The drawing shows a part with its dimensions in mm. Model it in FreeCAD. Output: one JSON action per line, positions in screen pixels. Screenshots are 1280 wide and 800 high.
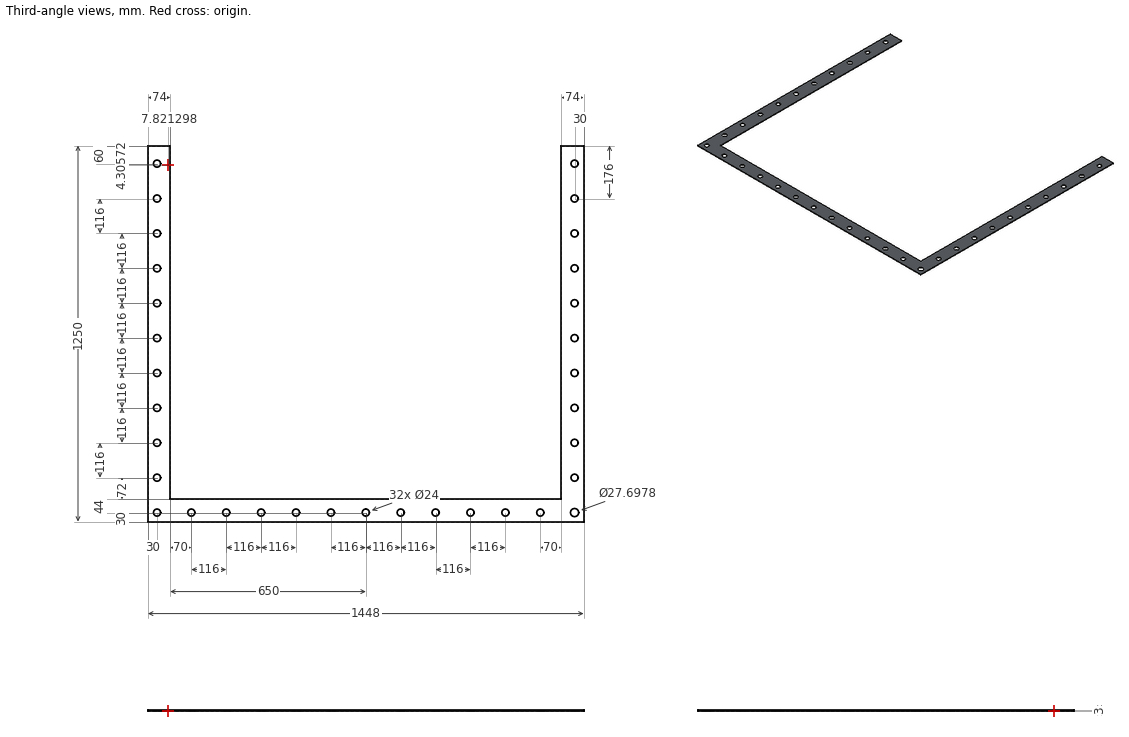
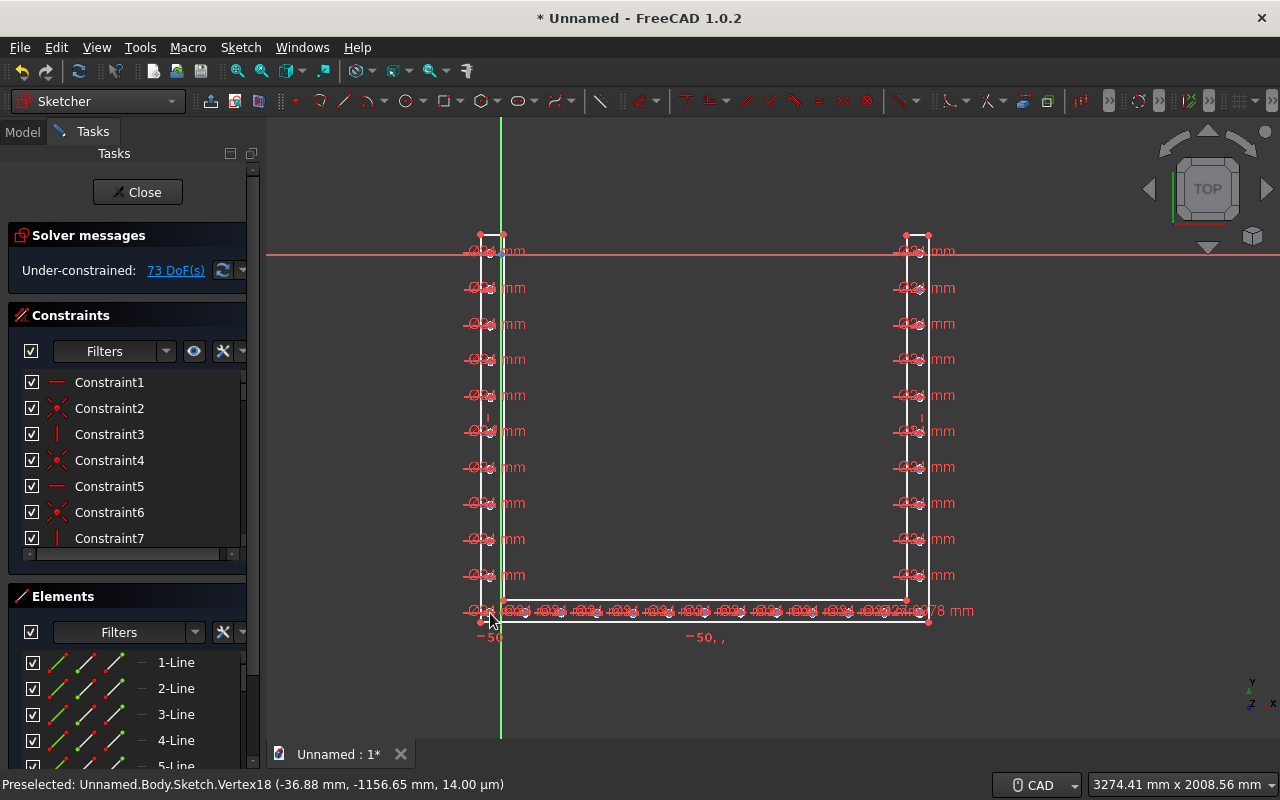
{"action": "left_click", "coordinate": [490, 577]}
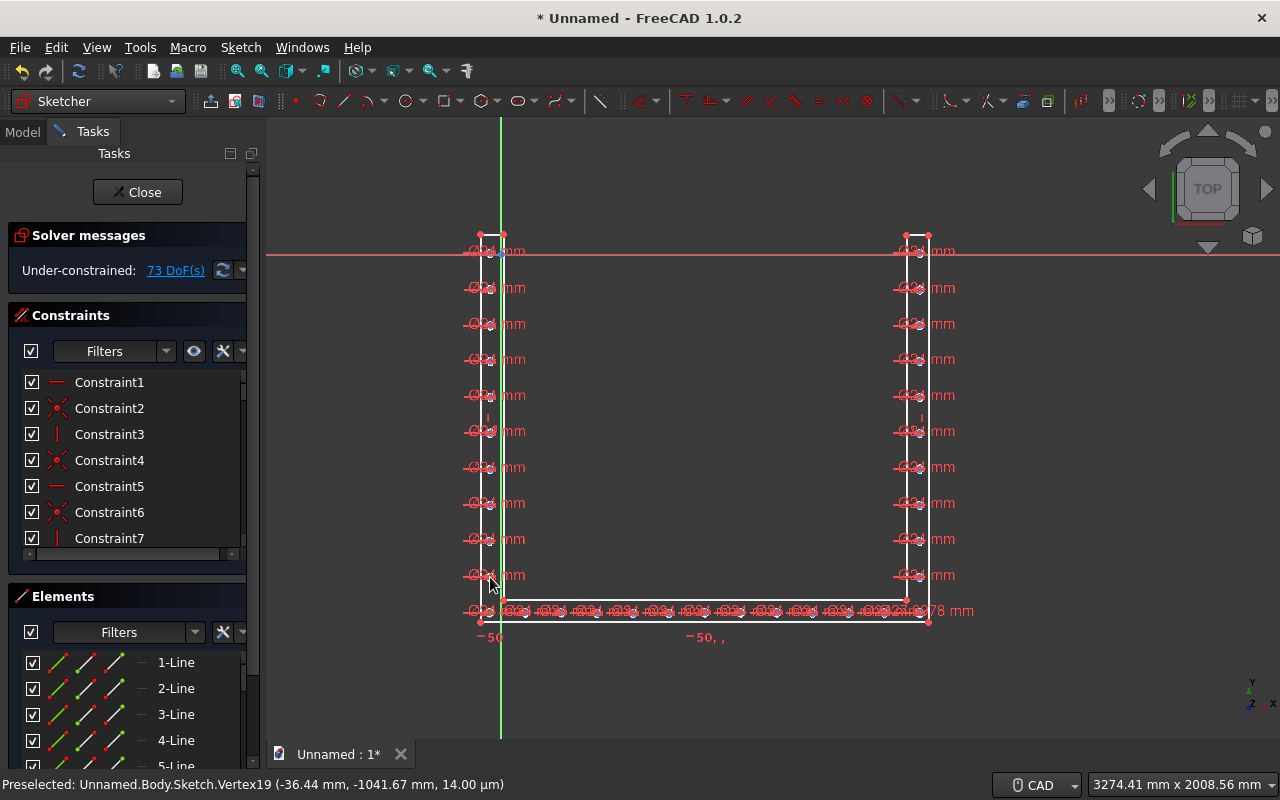
{"action": "left_click", "coordinate": [728, 102]}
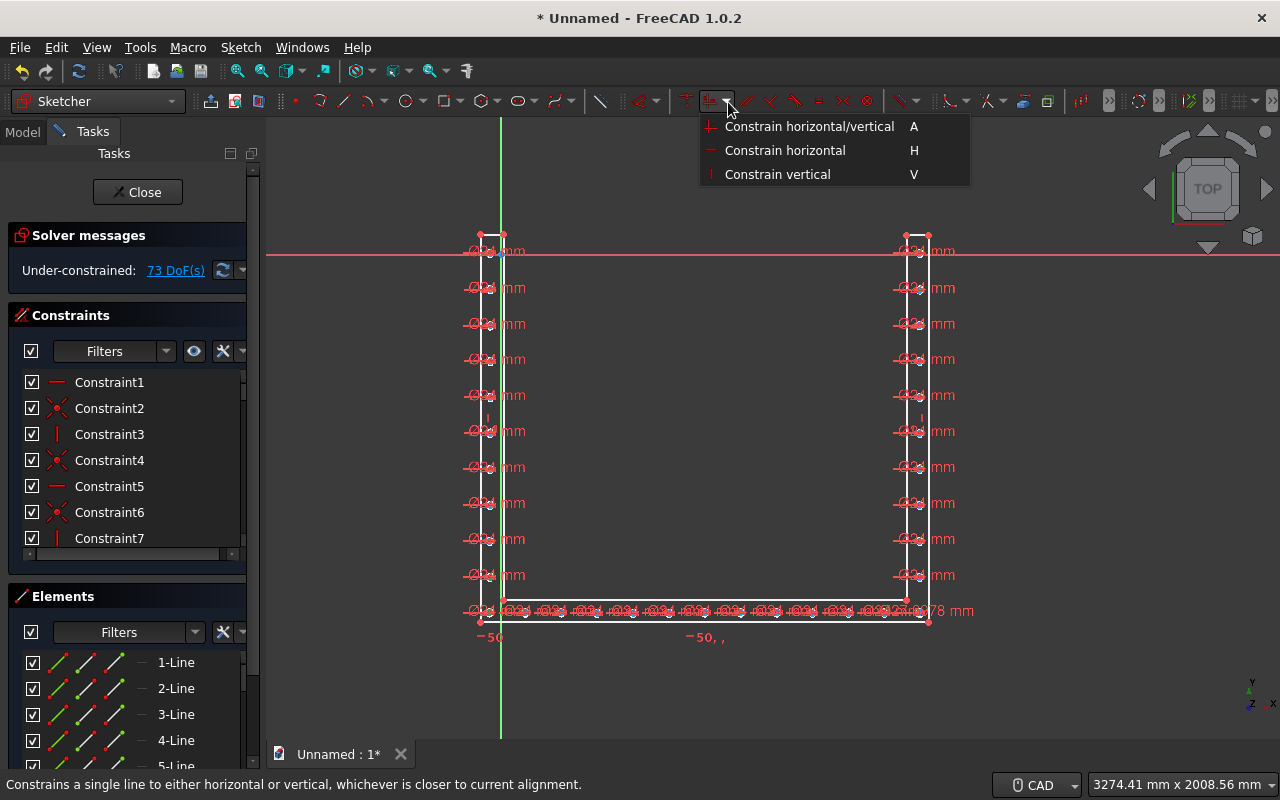
{"action": "left_click", "coordinate": [835, 174]}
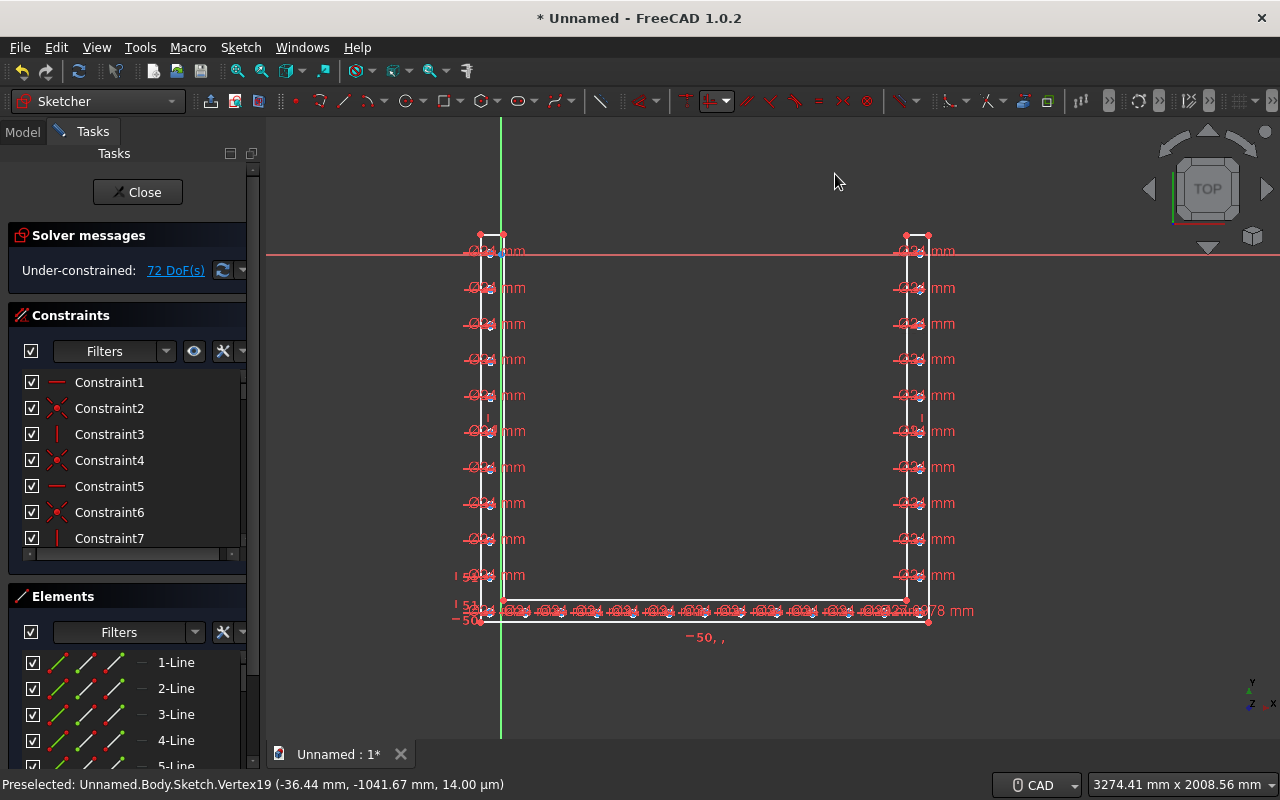
{"action": "left_click", "coordinate": [490, 613]}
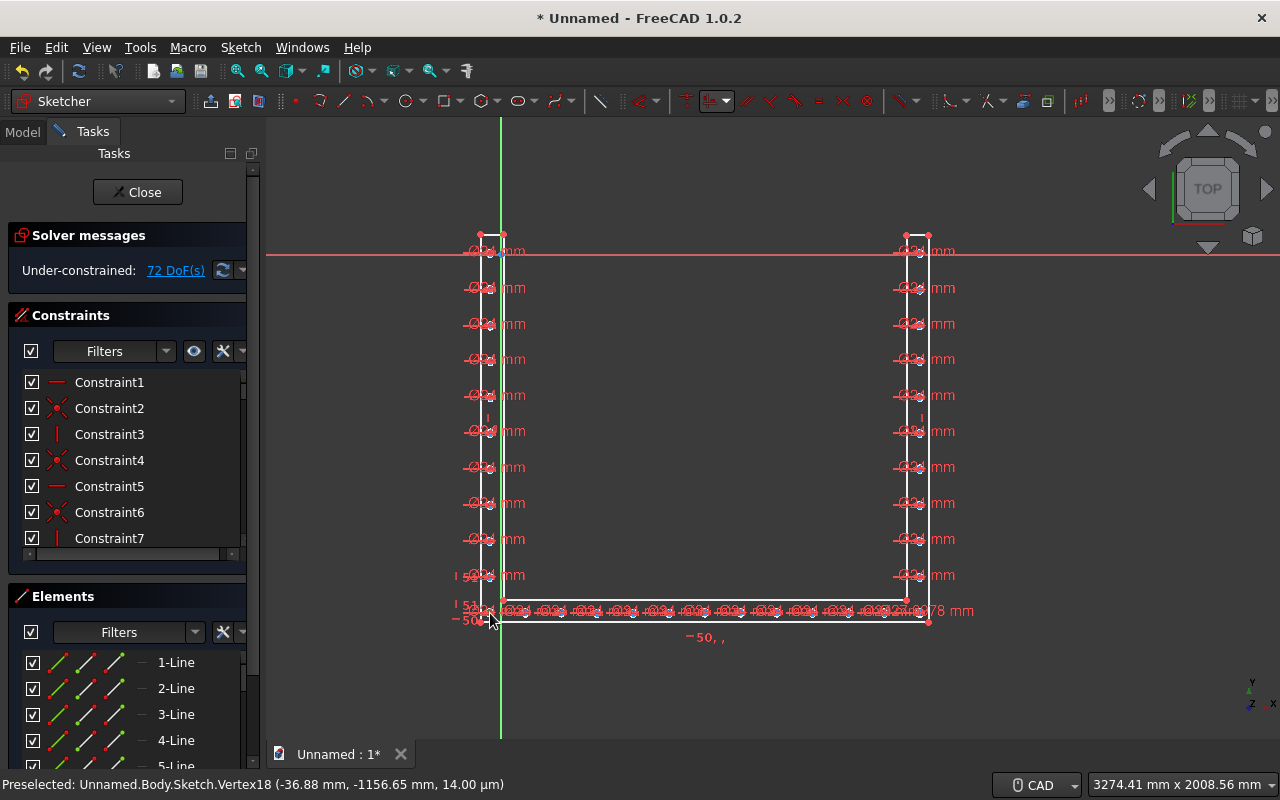
{"action": "left_click", "coordinate": [526, 613]}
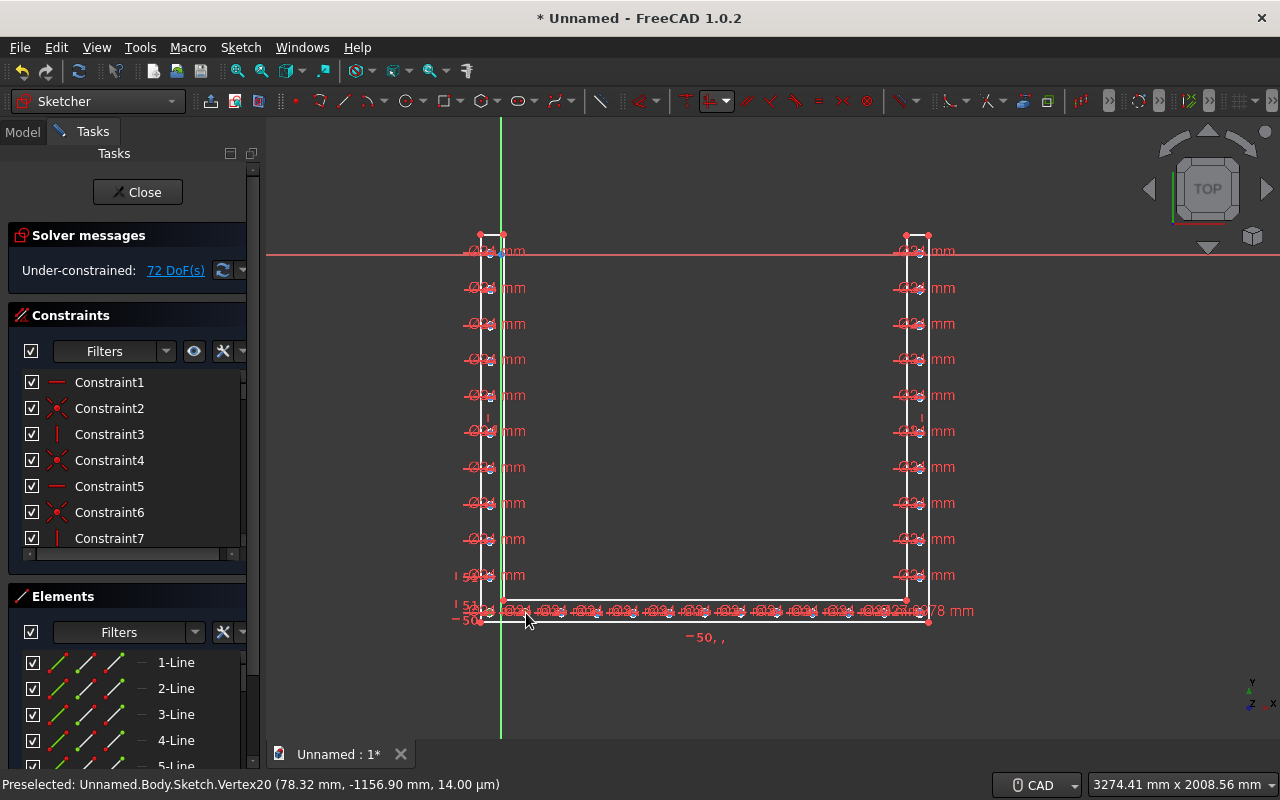
{"action": "left_click", "coordinate": [728, 102]}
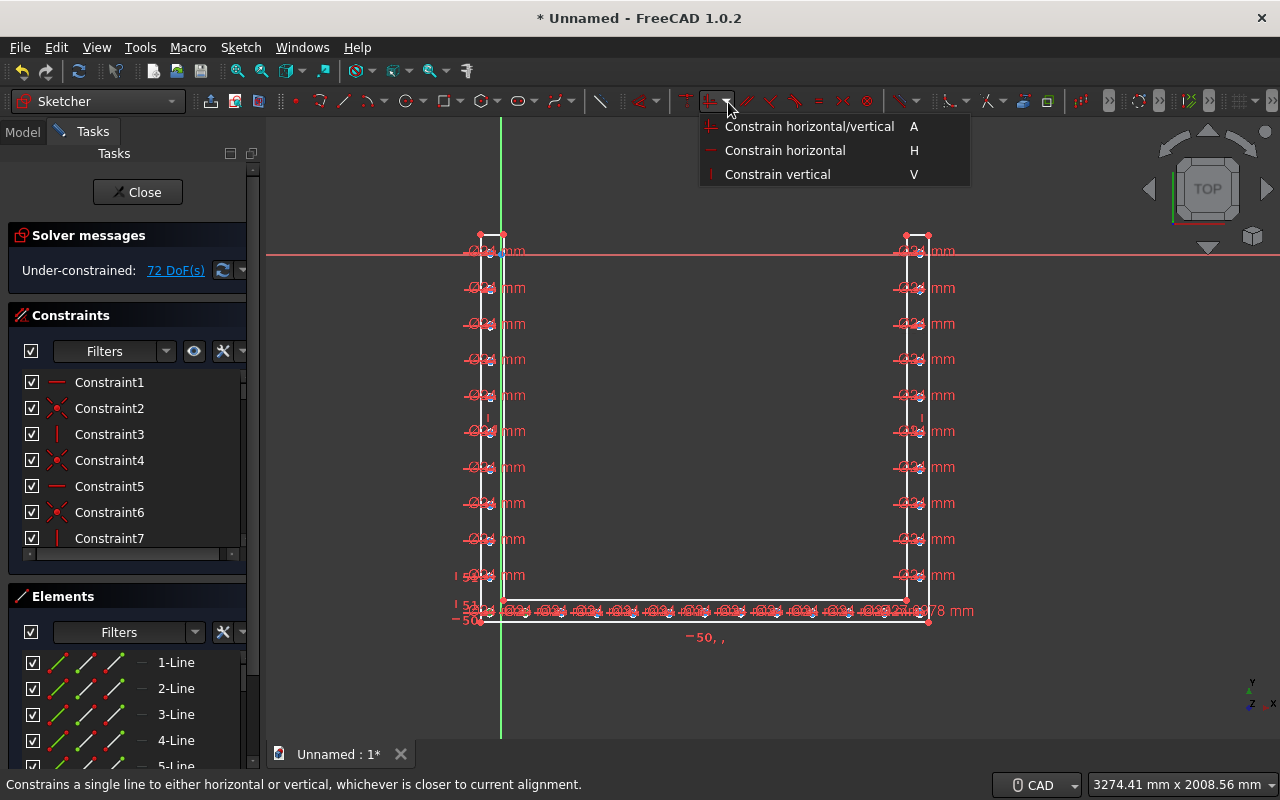
{"action": "left_click", "coordinate": [835, 150]}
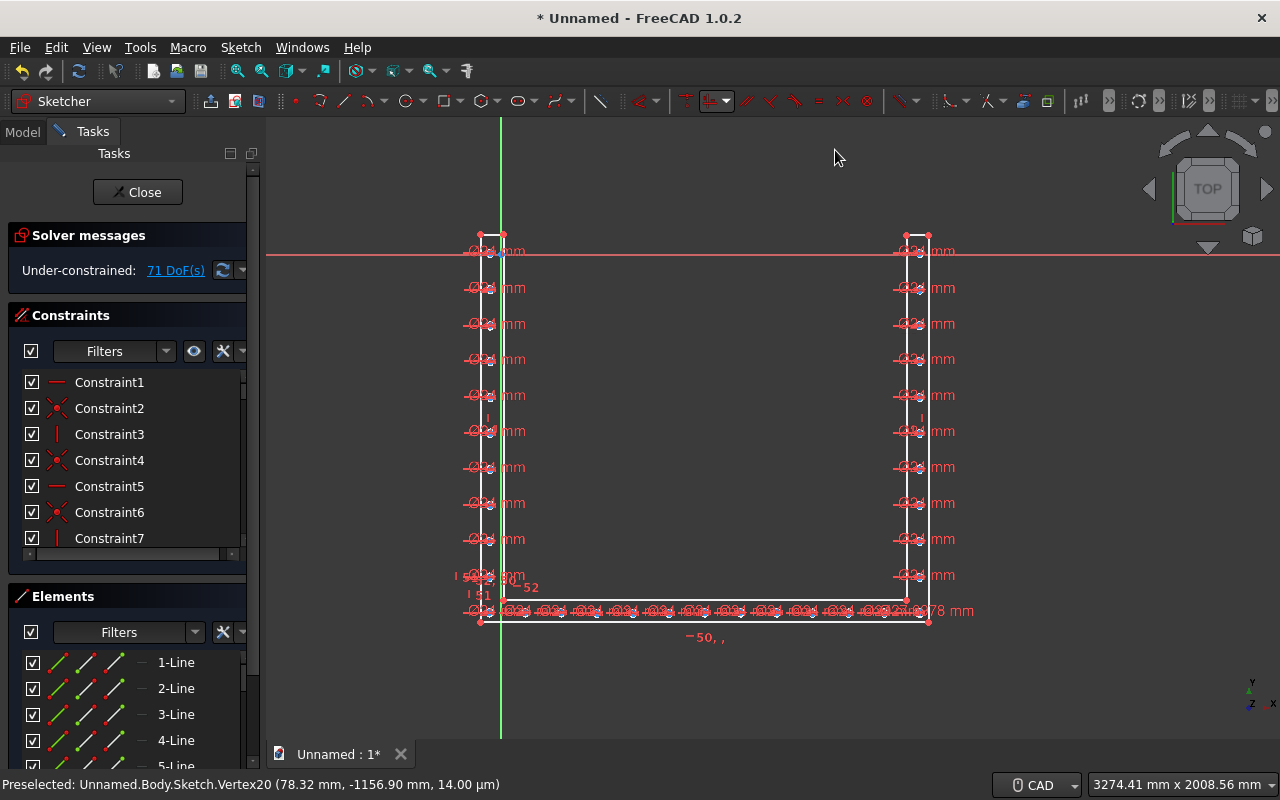
{"action": "left_click", "coordinate": [490, 577]}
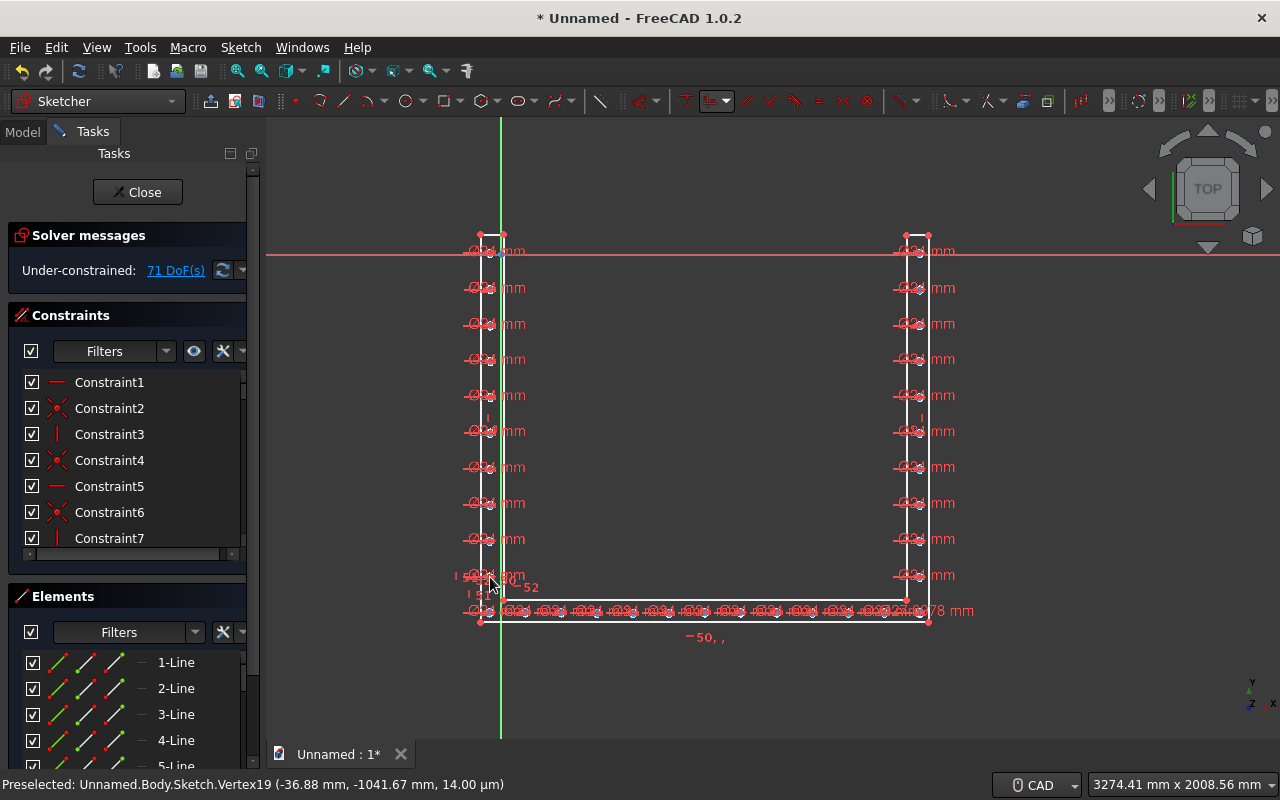
{"action": "left_click", "coordinate": [490, 541]}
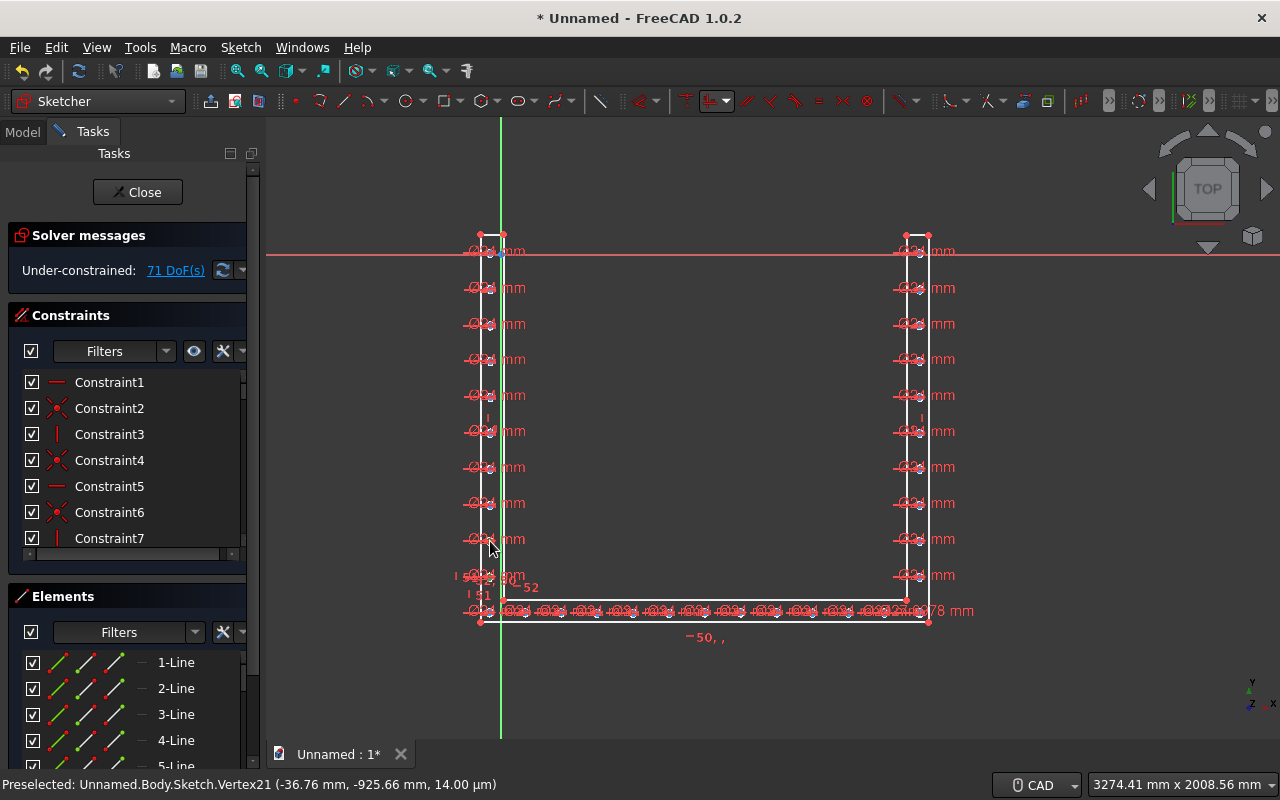
{"action": "key", "text": "v"}